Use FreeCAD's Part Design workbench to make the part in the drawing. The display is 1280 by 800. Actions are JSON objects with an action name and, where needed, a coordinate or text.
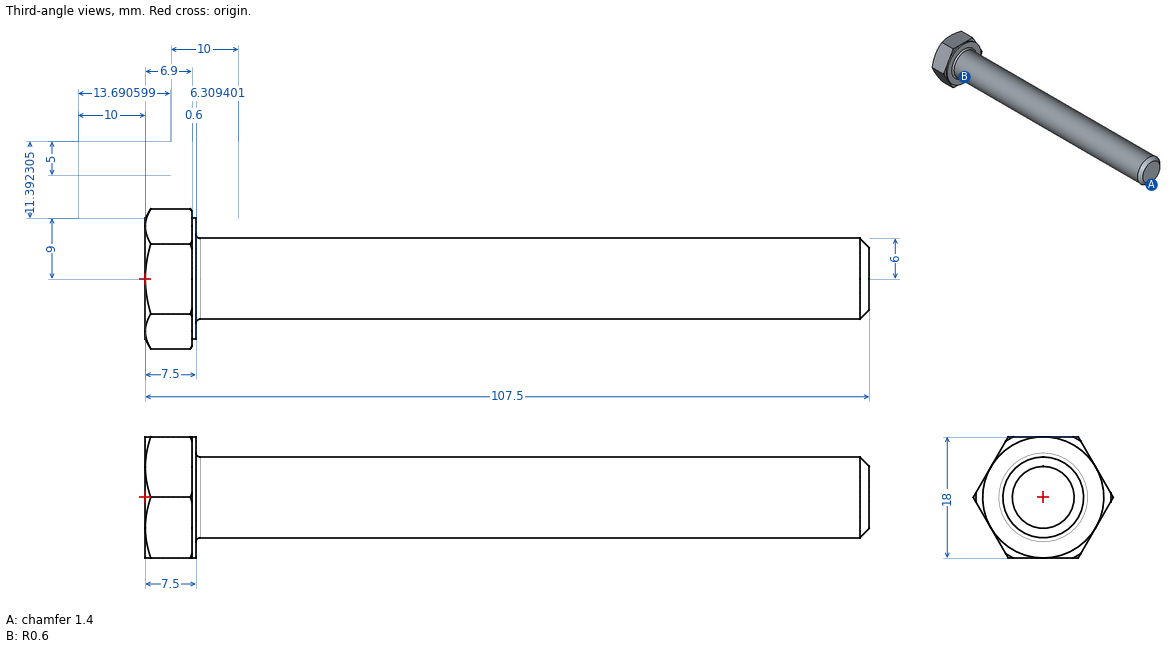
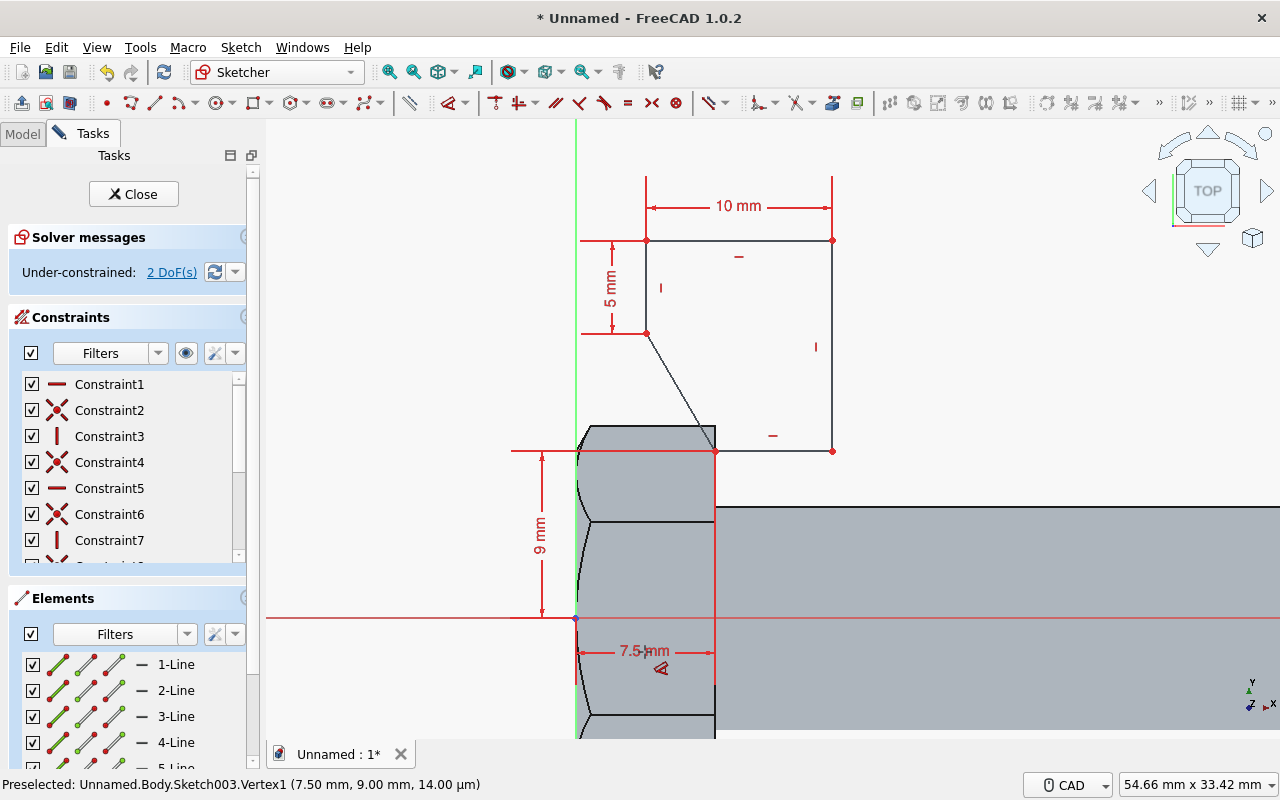
{"action": "left_click", "coordinate": [750, 451]}
{"action": "left_click", "coordinate": [774, 485]}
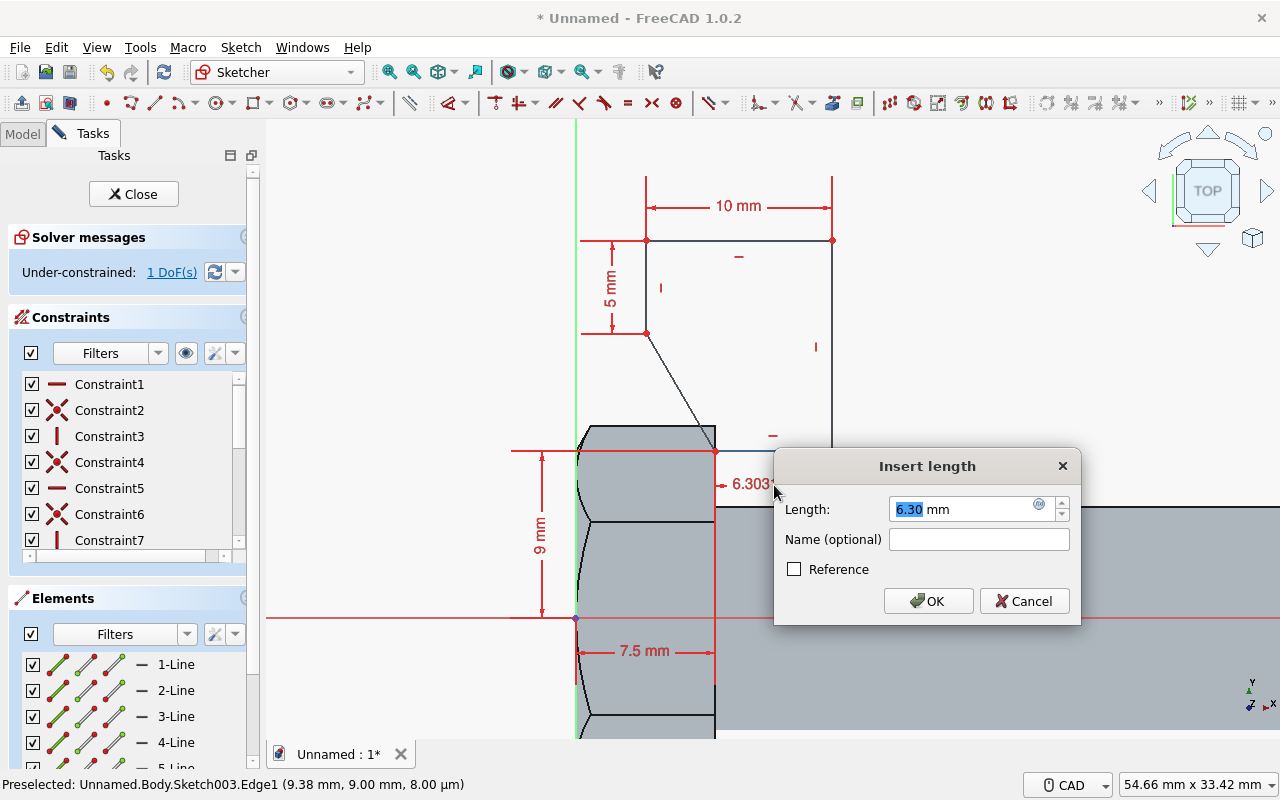
{"action": "type", "text": "6.309401"}
{"action": "key", "text": "Return"}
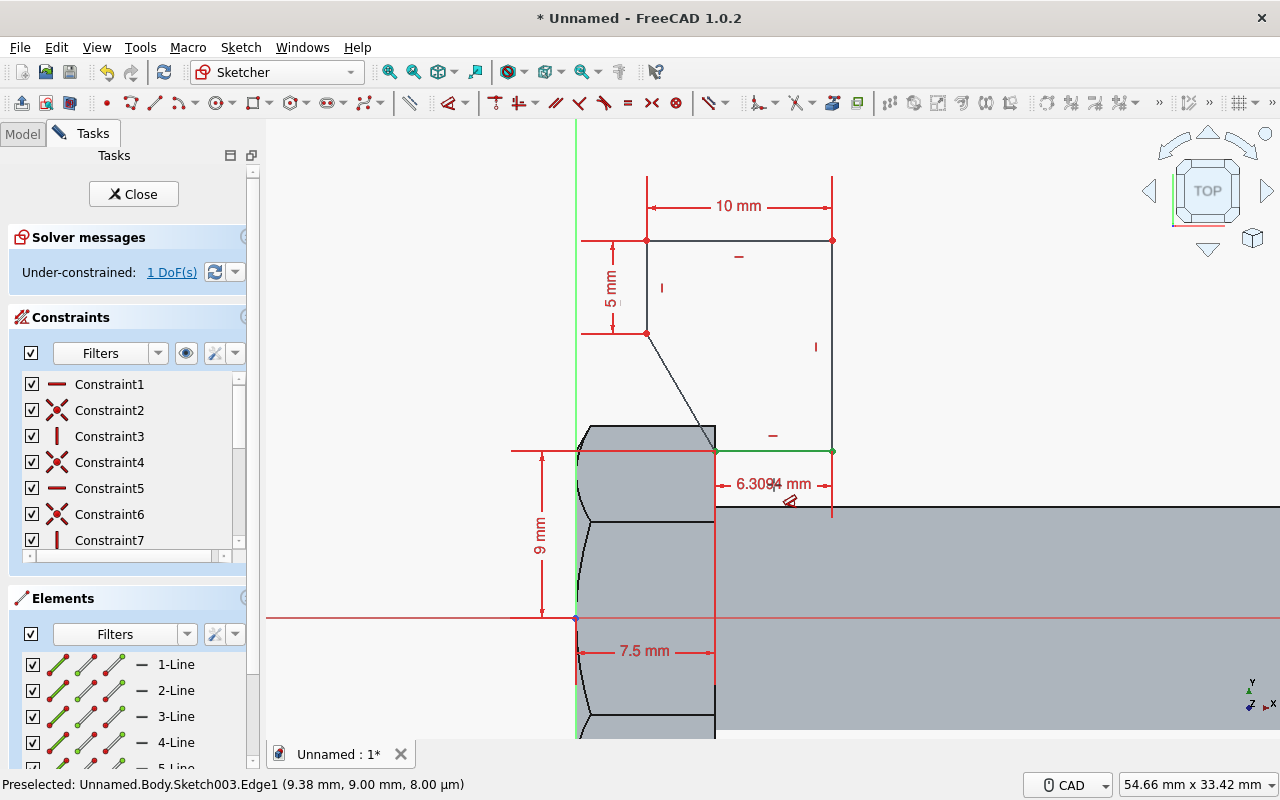
{"action": "left_click", "coordinate": [832, 388]}
{"action": "left_click", "coordinate": [866, 346]}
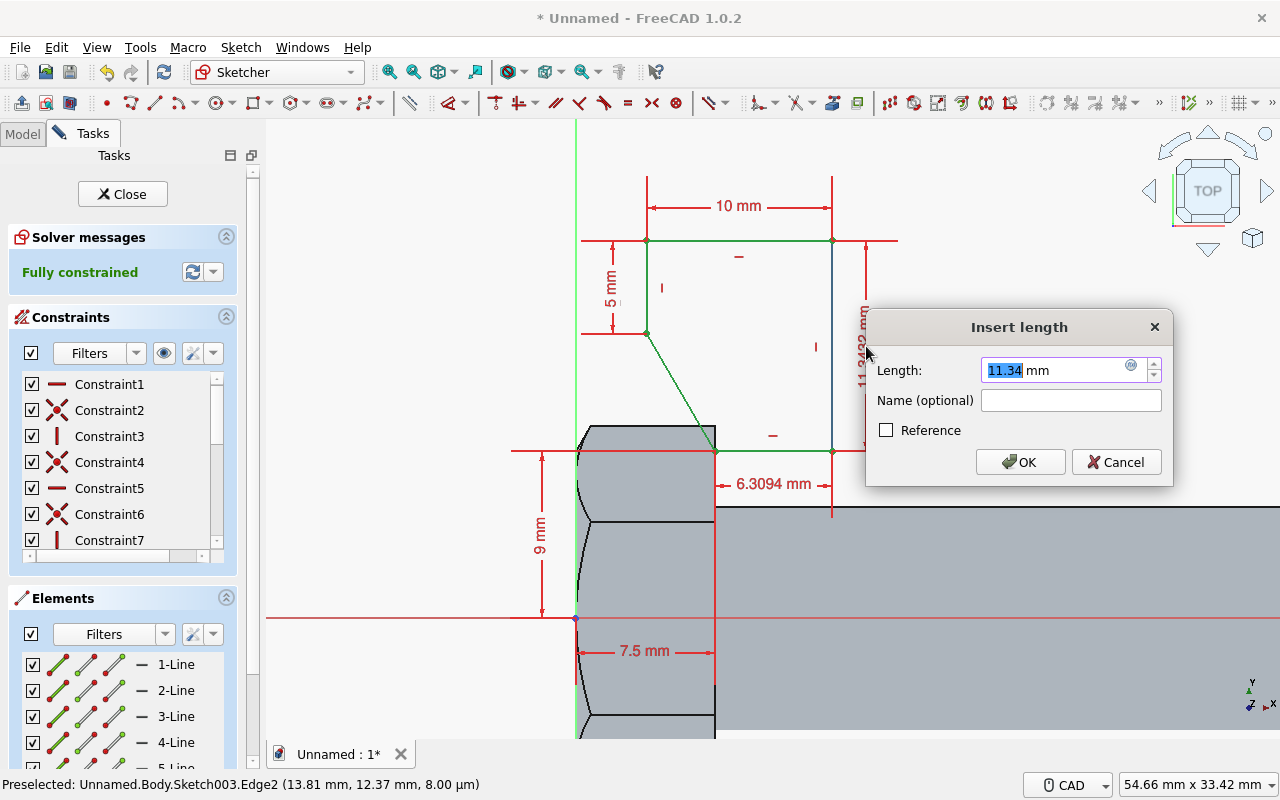
{"action": "type", "text": "11.392305"}
{"action": "key", "text": "Return"}
{"action": "key", "text": "Escape"}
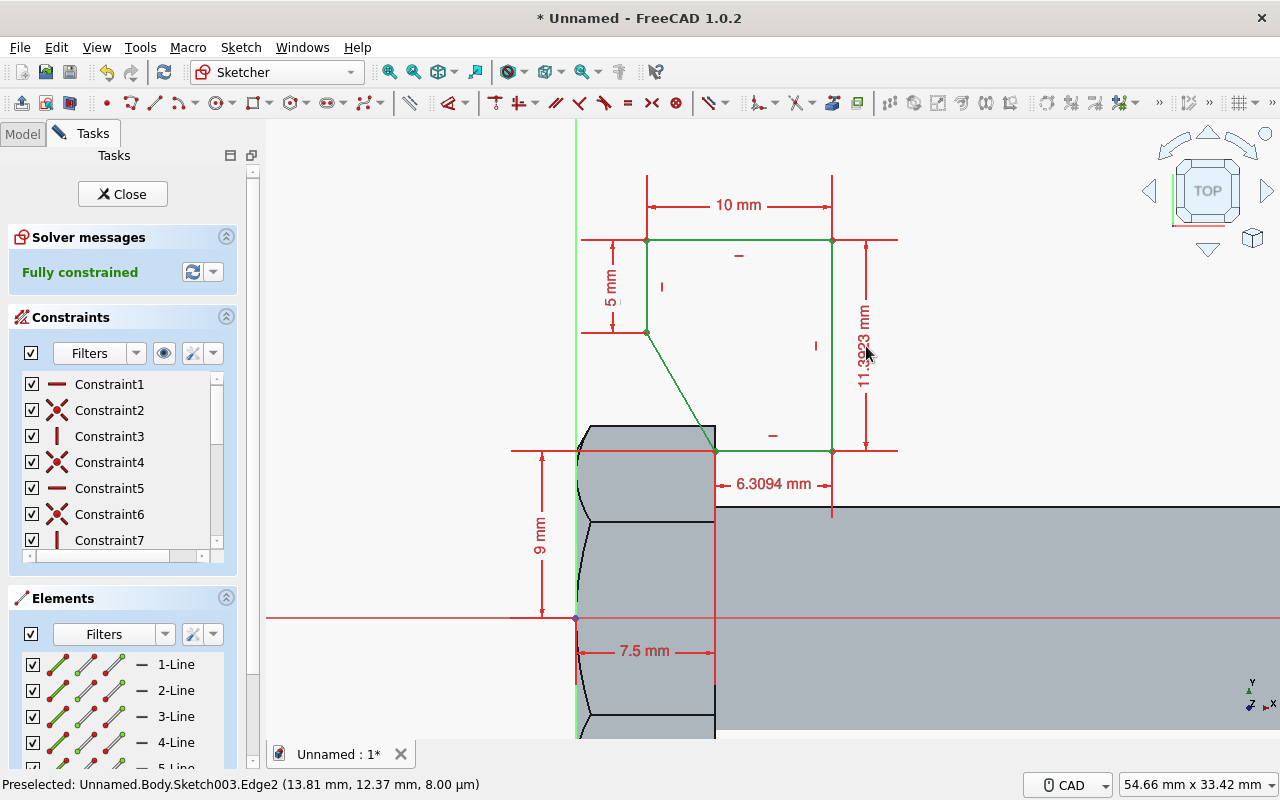
{"action": "left_click", "coordinate": [123, 194]}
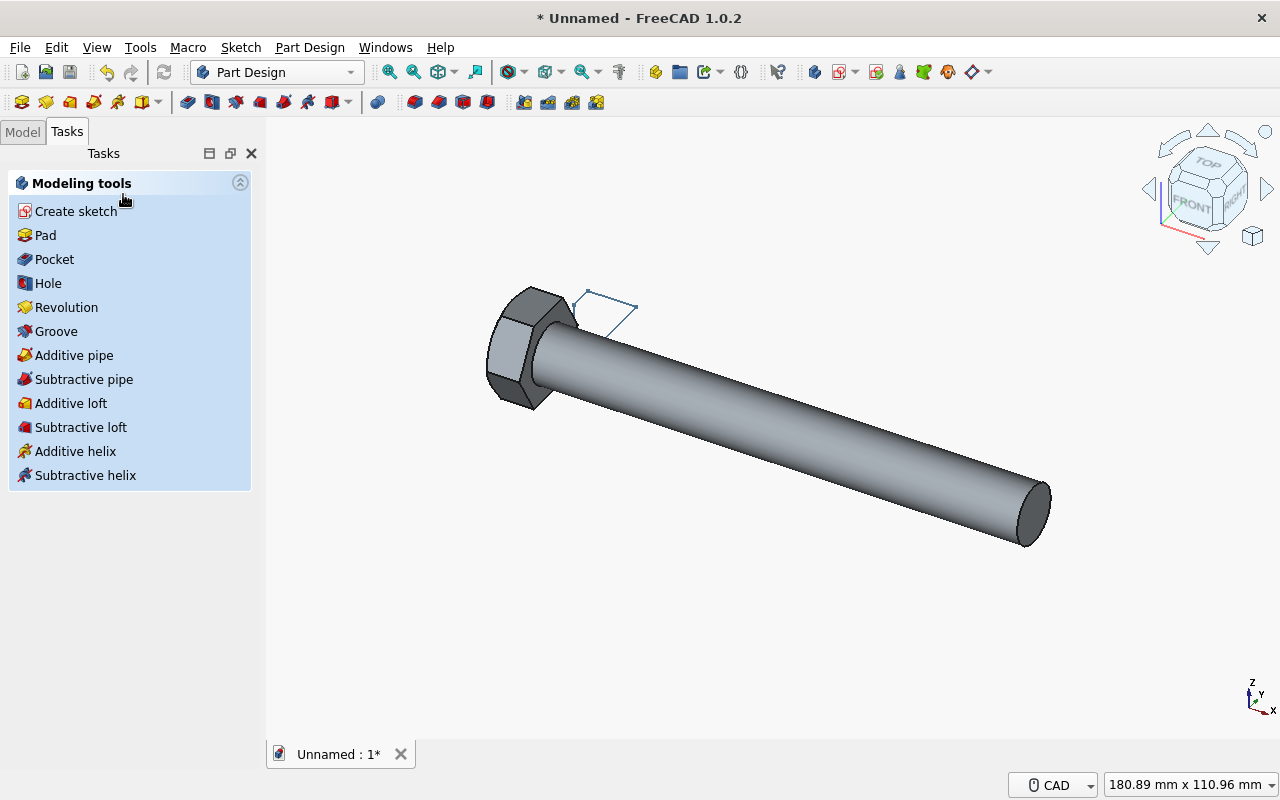
{"action": "left_click", "coordinate": [236, 102]}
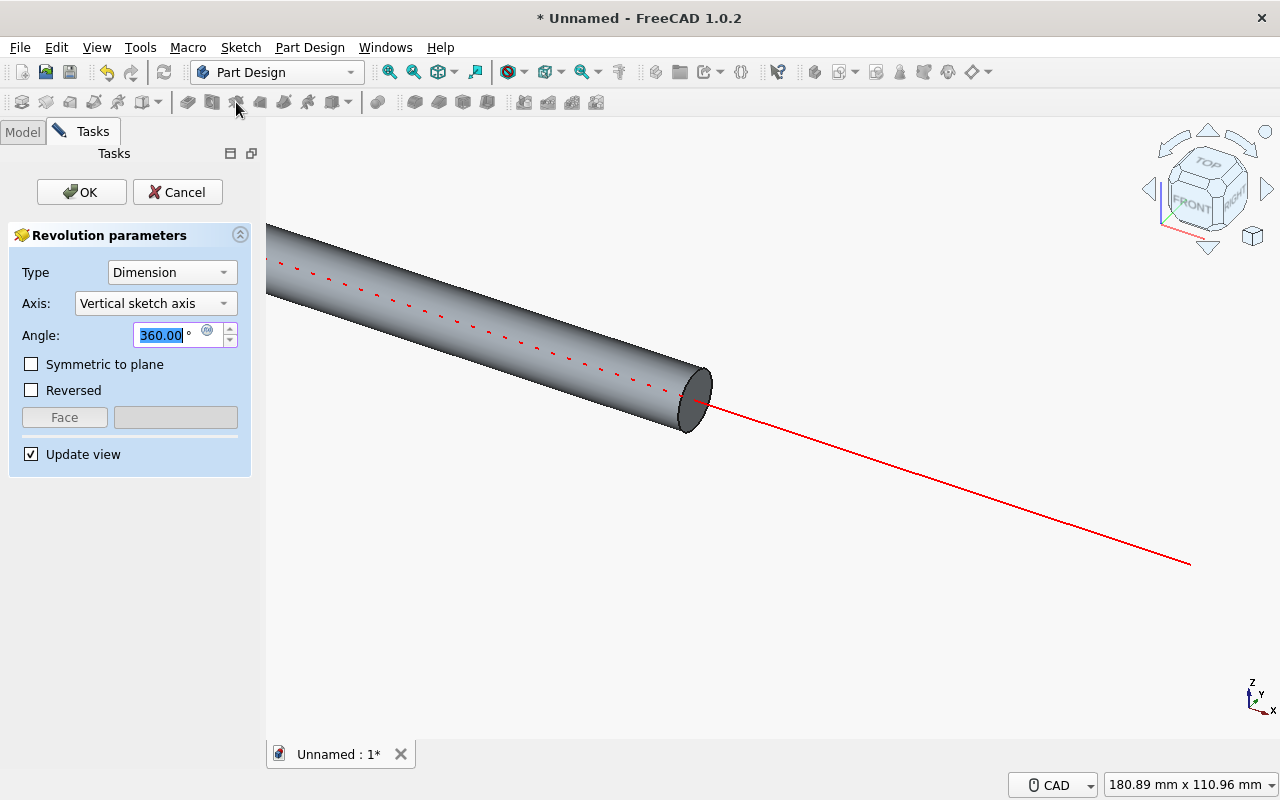
{"action": "left_click", "coordinate": [156, 304]}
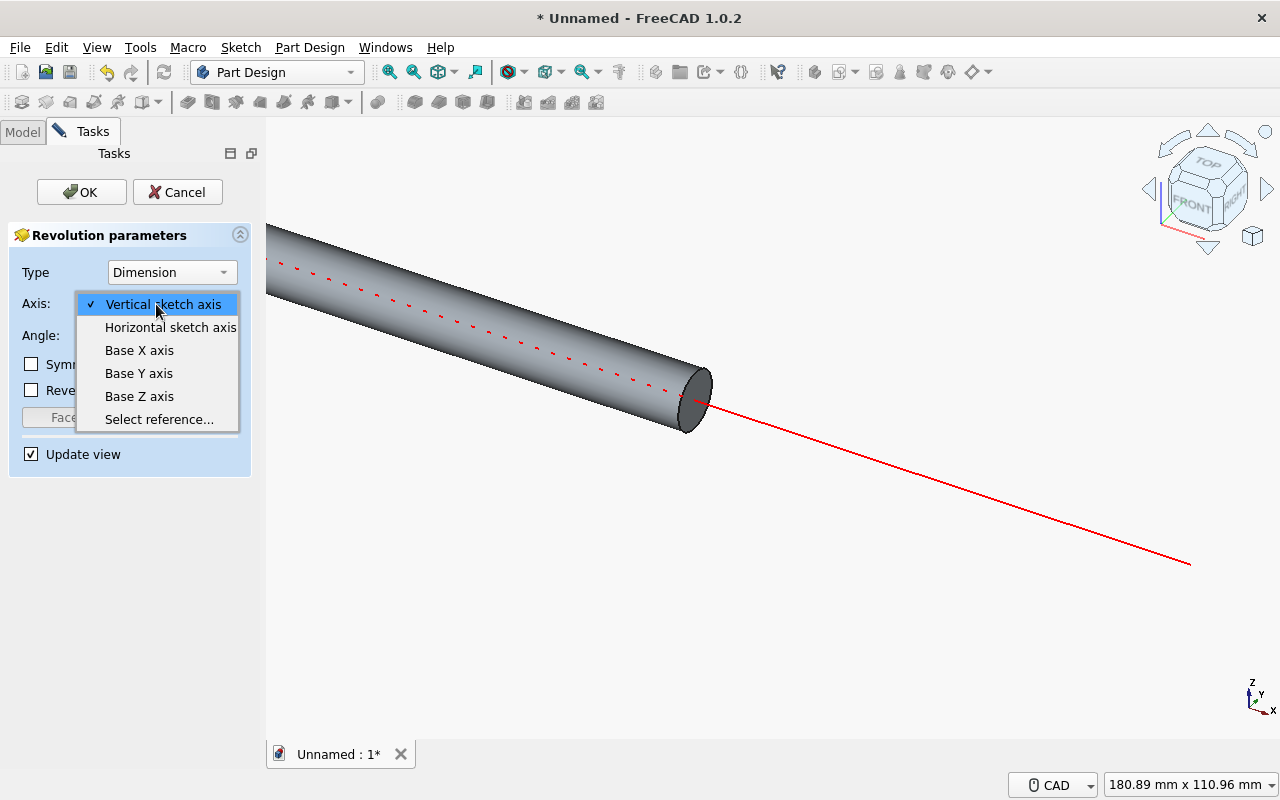
{"action": "left_click", "coordinate": [156, 328]}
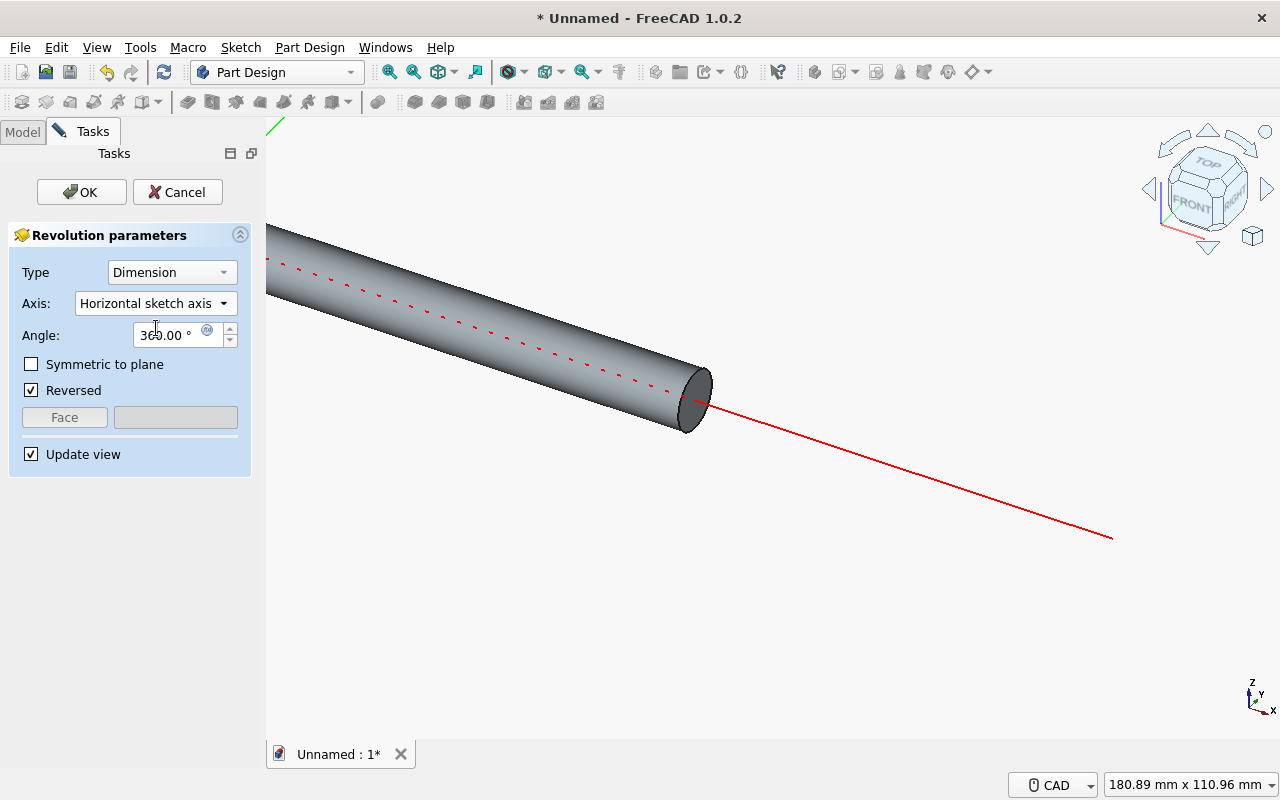
{"action": "left_click", "coordinate": [82, 192]}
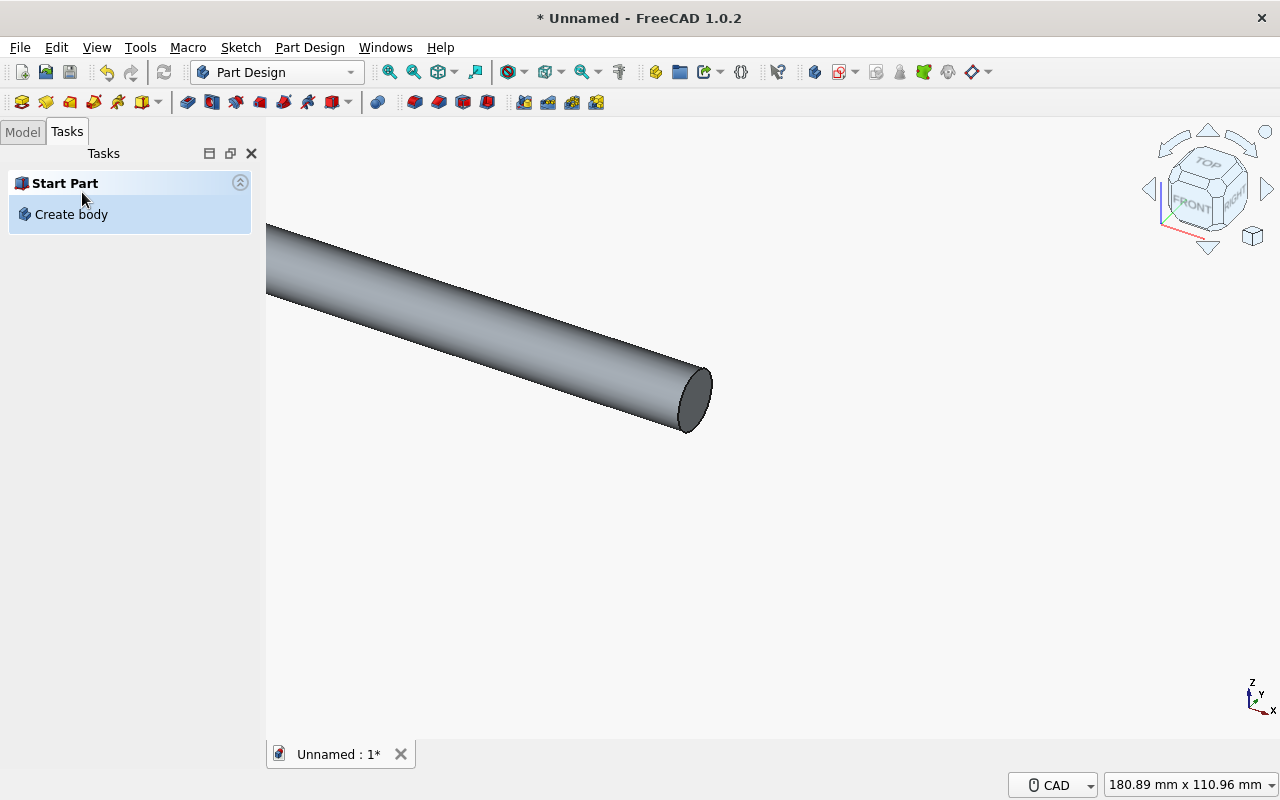
{"action": "key", "text": "v f"}